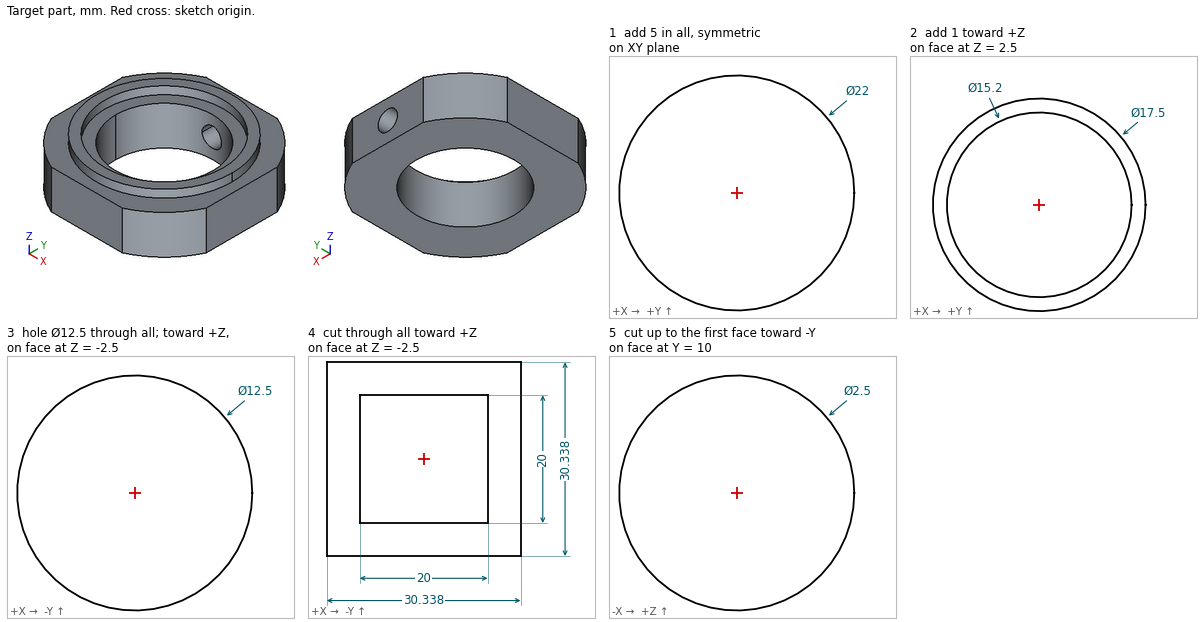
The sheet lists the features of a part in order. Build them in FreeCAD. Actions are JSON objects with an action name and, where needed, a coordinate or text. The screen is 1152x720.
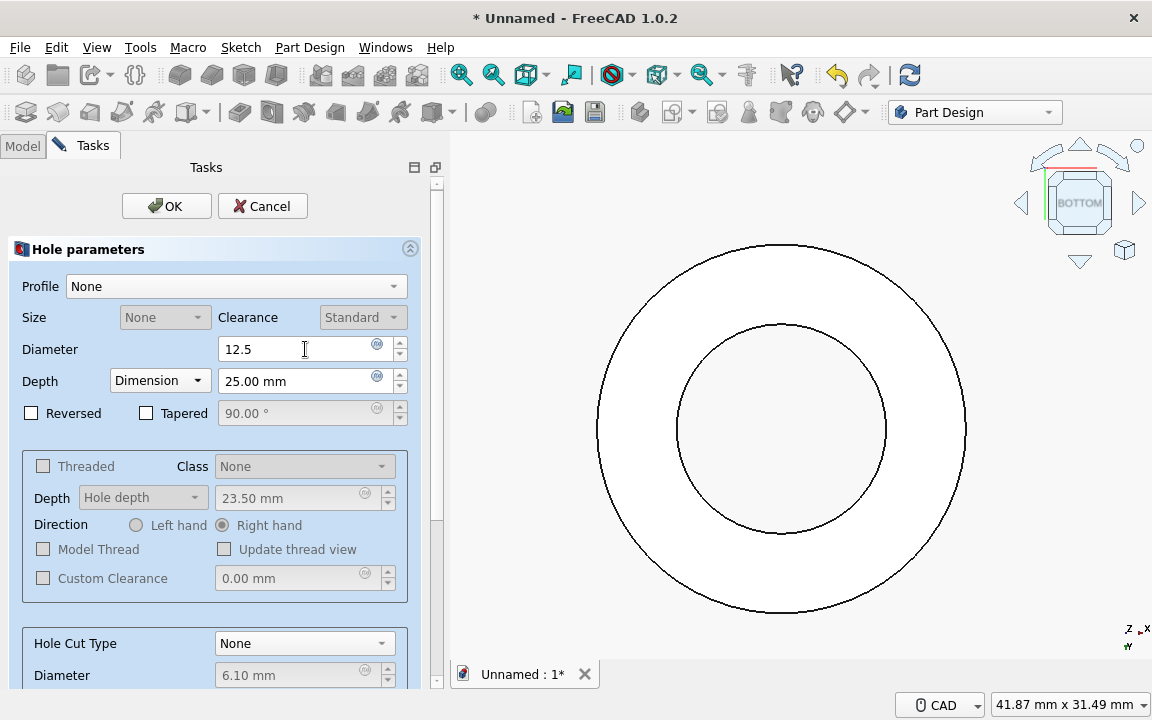
{"action": "left_click", "coordinate": [161, 380]}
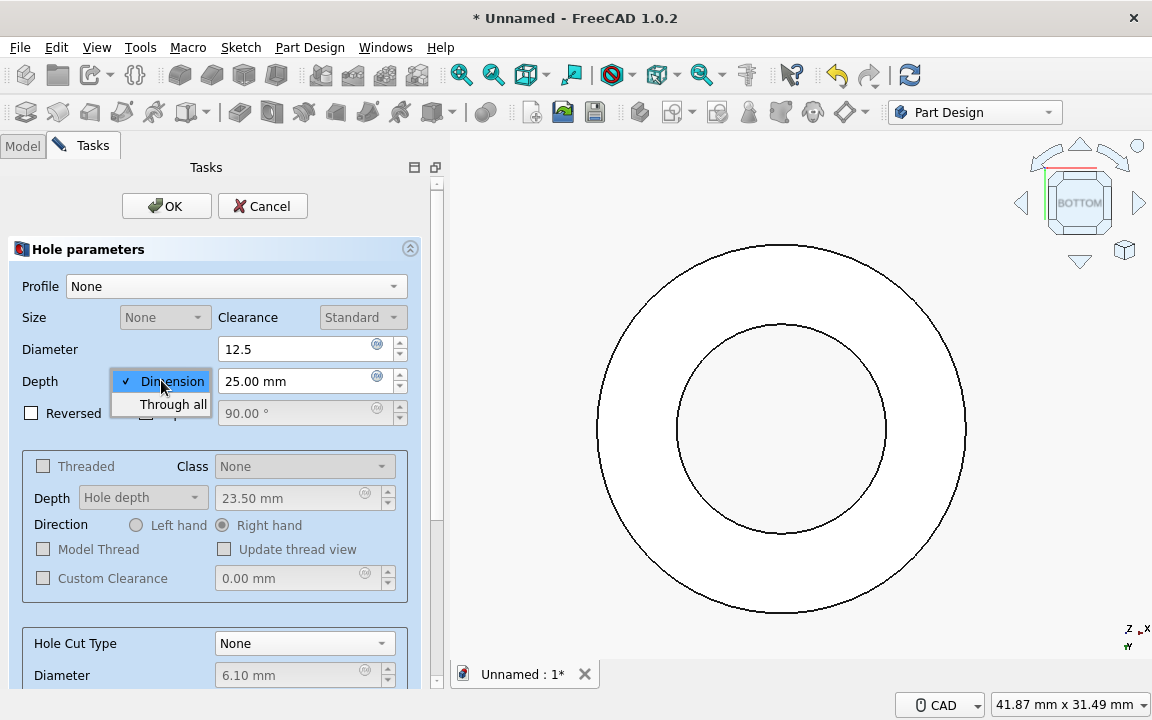
{"action": "left_click", "coordinate": [160, 404]}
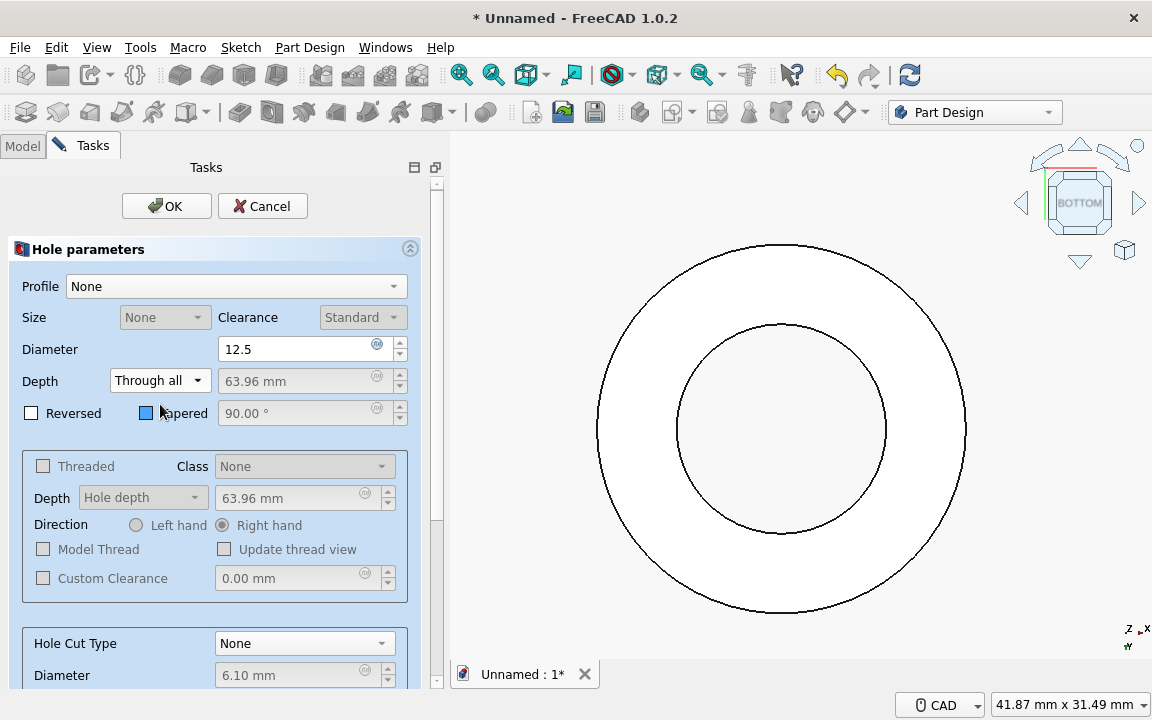
{"action": "left_click", "coordinate": [167, 206]}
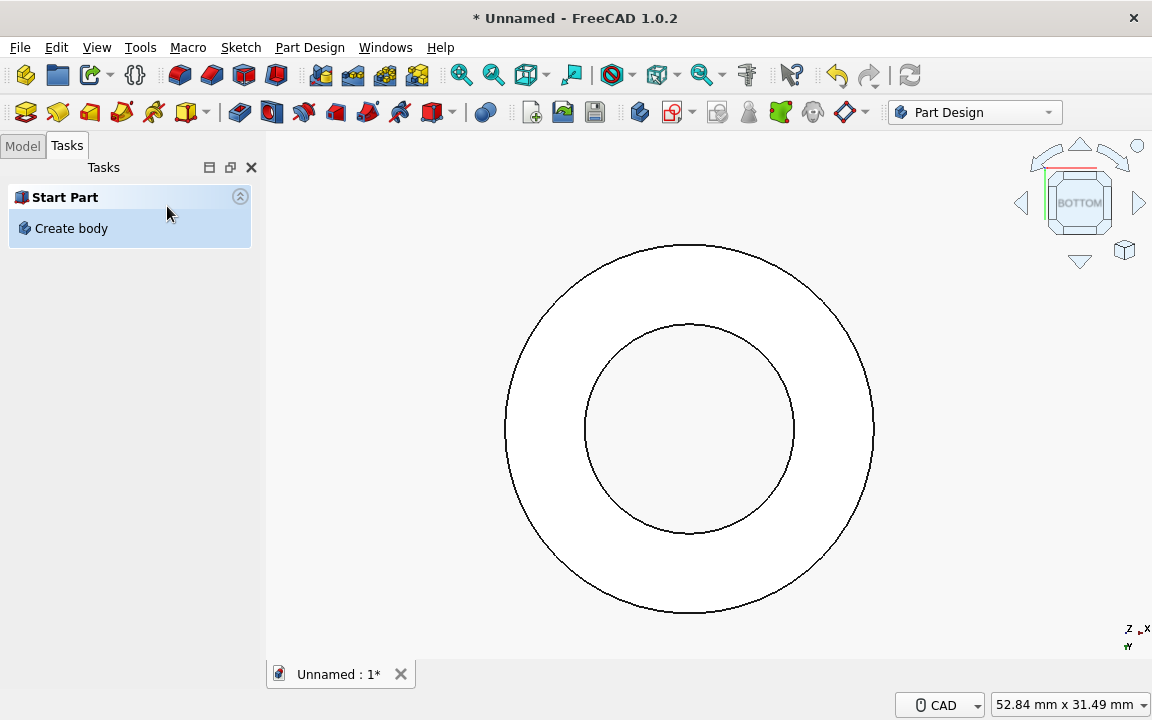
{"action": "left_click", "coordinate": [795, 533]}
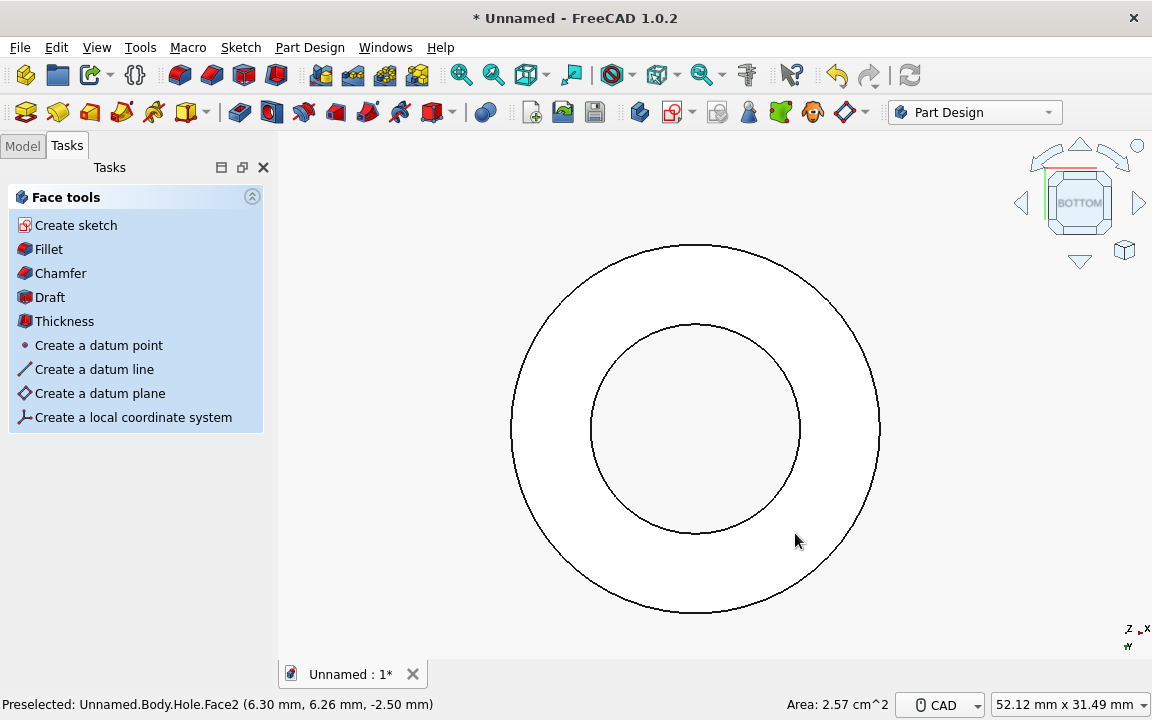
{"action": "left_click", "coordinate": [672, 112]}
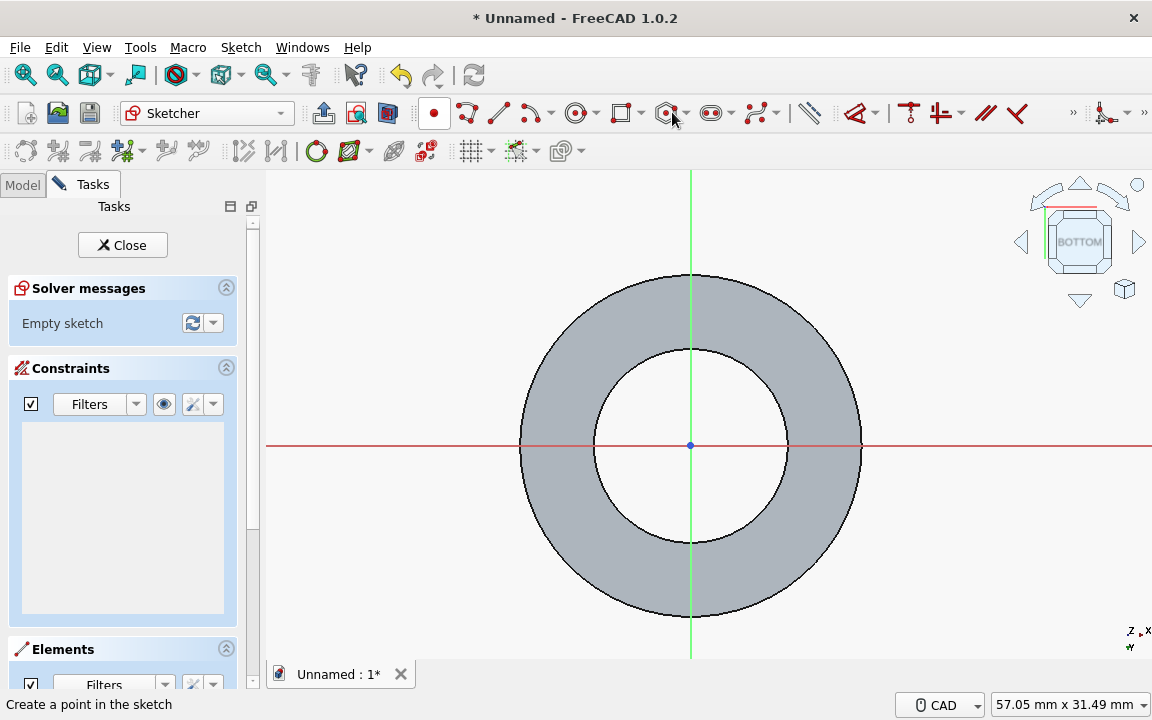
{"action": "scroll", "coordinate": [538, 350], "scroll_direction": "down", "scroll_amount": 2}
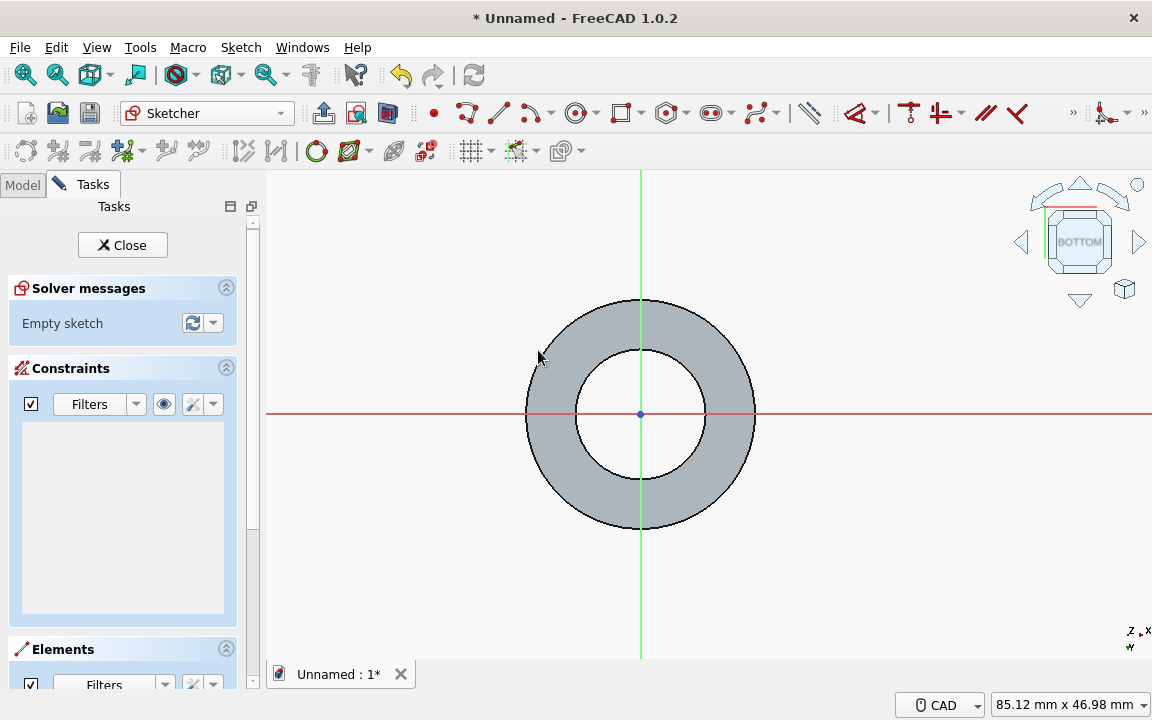
{"action": "key", "text": "g v"}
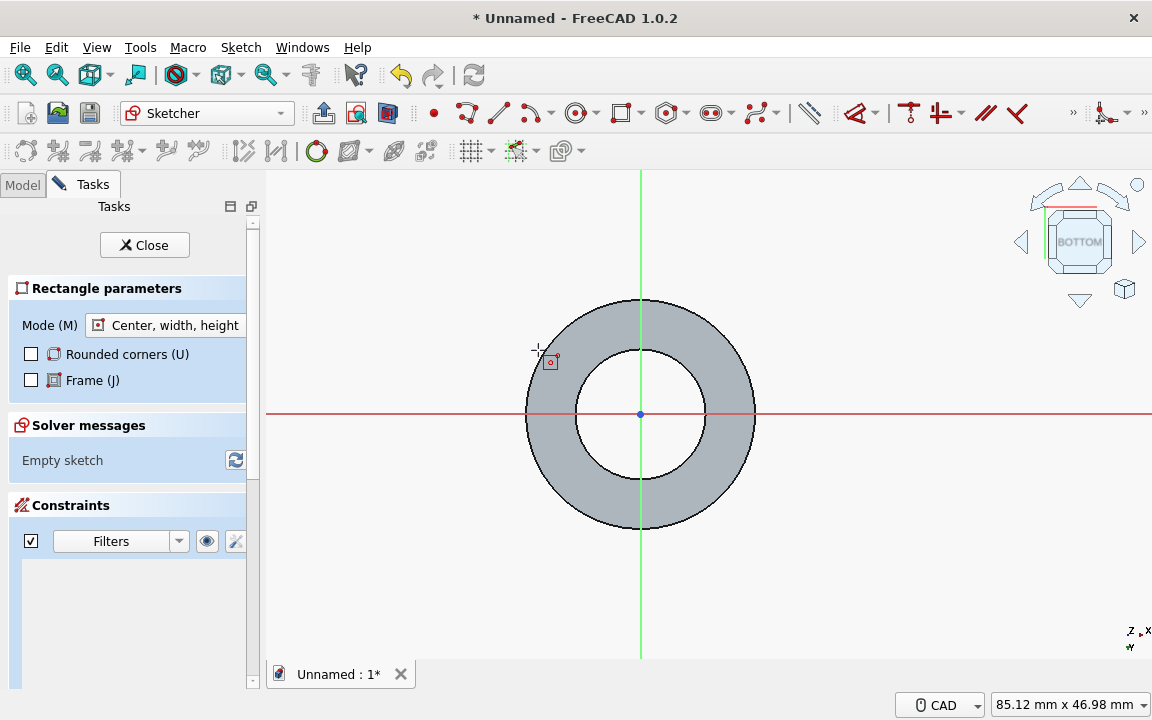
{"action": "left_click", "coordinate": [641, 414]}
{"action": "mouse_move", "coordinate": [798, 257]}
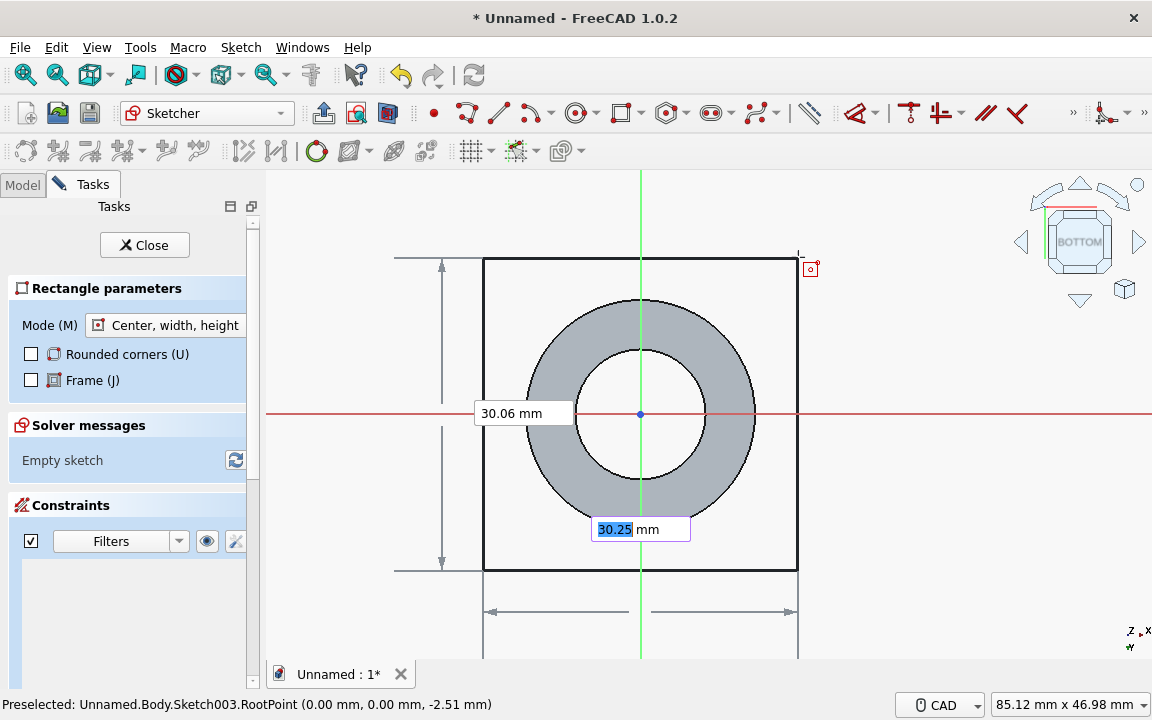
{"action": "type", "text": "30.338"}
{"action": "key", "text": "Tab"}
{"action": "type", "text": "30.338"}
{"action": "key", "text": "Return"}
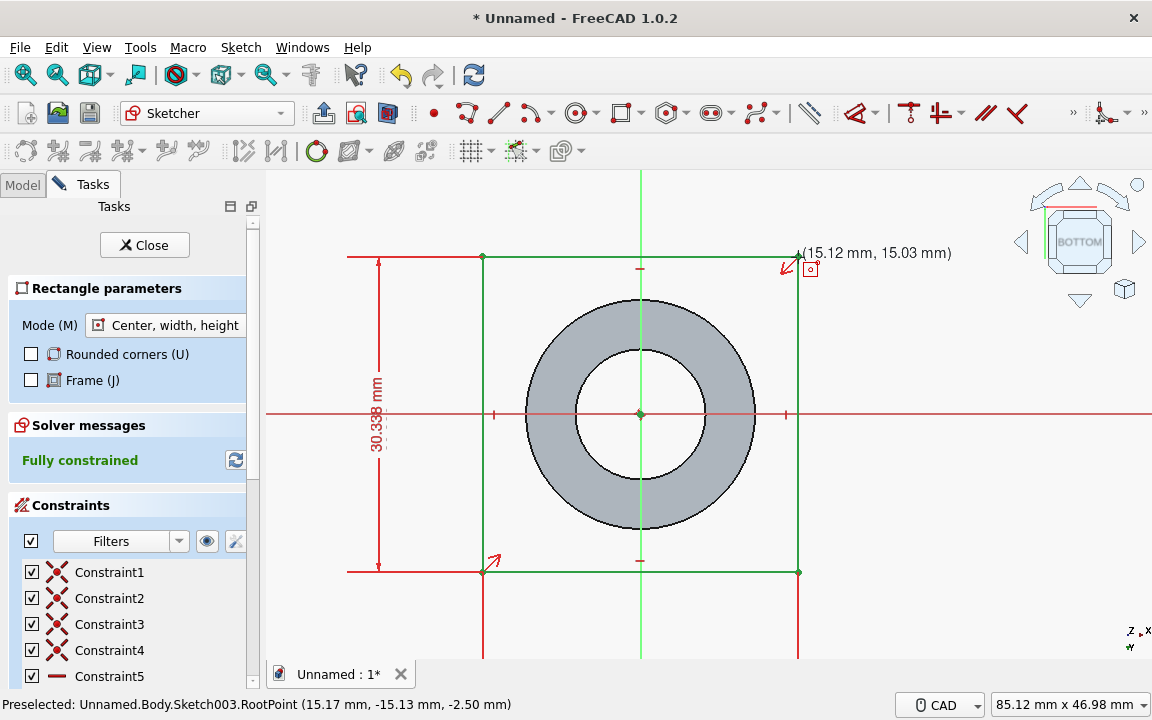
{"action": "left_click", "coordinate": [641, 414]}
{"action": "mouse_move", "coordinate": [745, 310]}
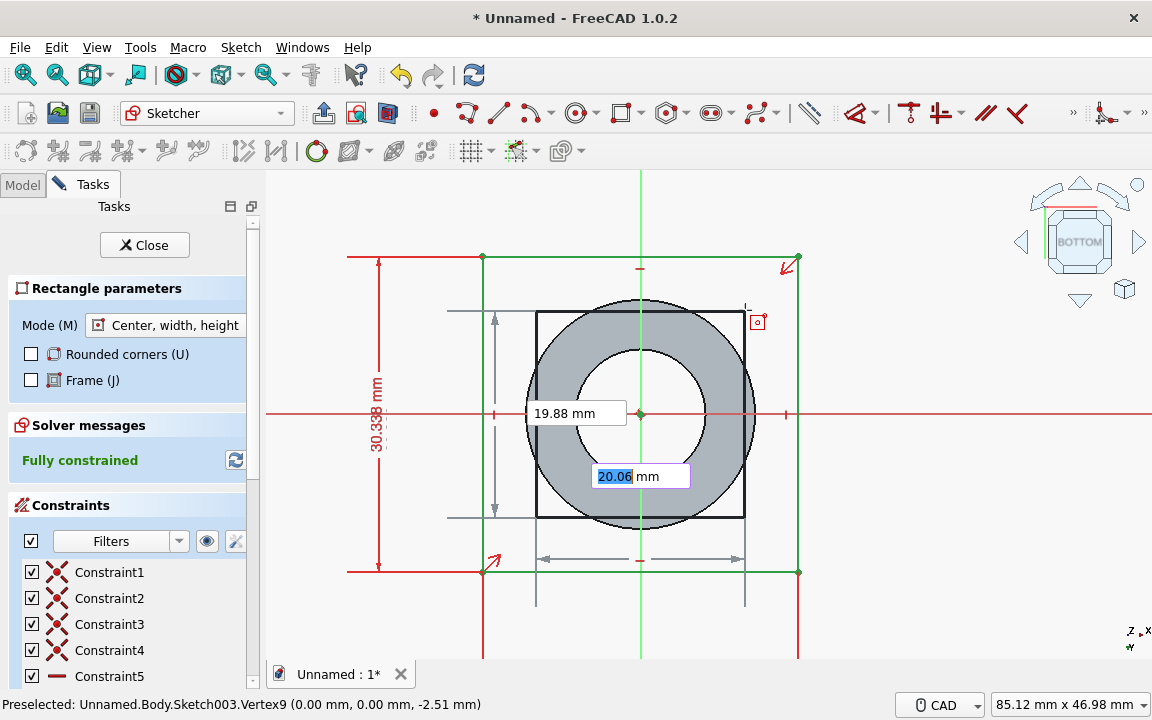
{"action": "type", "text": "20"}
{"action": "key", "text": "Tab"}
{"action": "type", "text": "20"}
{"action": "key", "text": "Return"}
{"action": "key", "text": "Escape"}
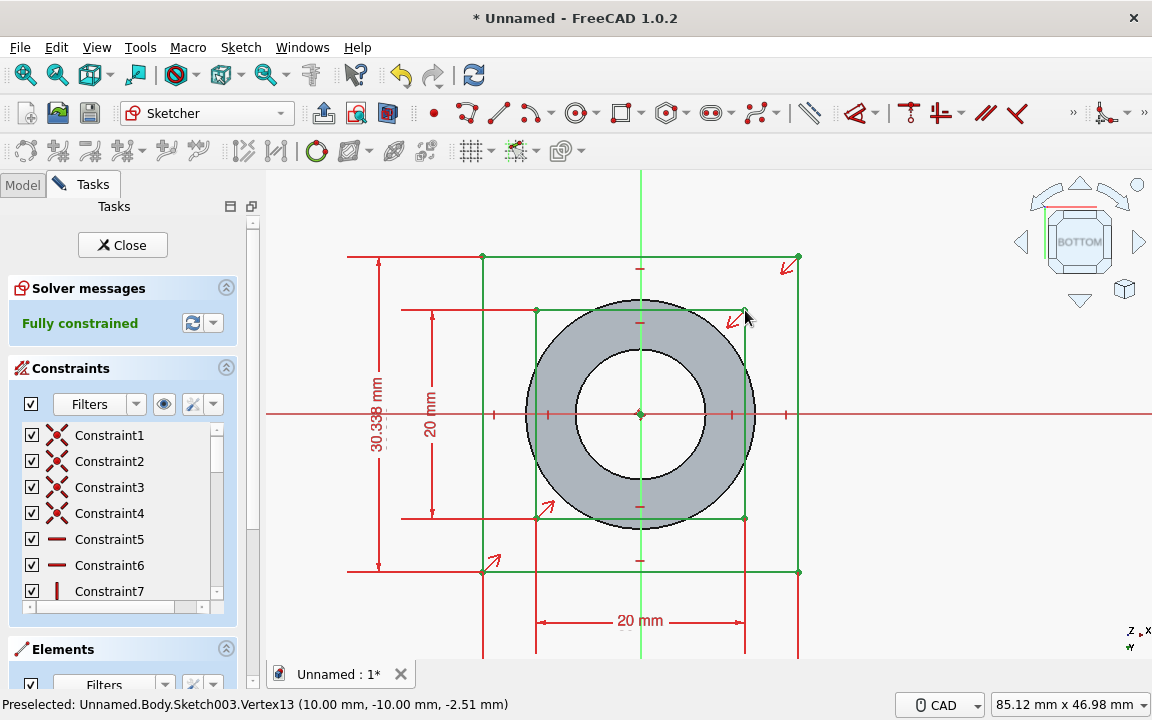
{"action": "left_click", "coordinate": [123, 245]}